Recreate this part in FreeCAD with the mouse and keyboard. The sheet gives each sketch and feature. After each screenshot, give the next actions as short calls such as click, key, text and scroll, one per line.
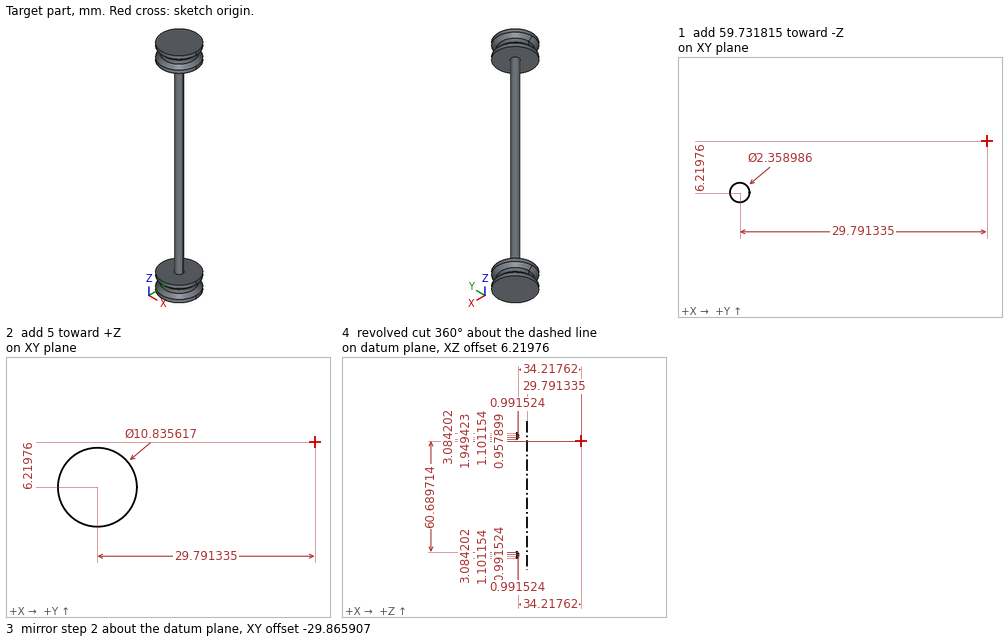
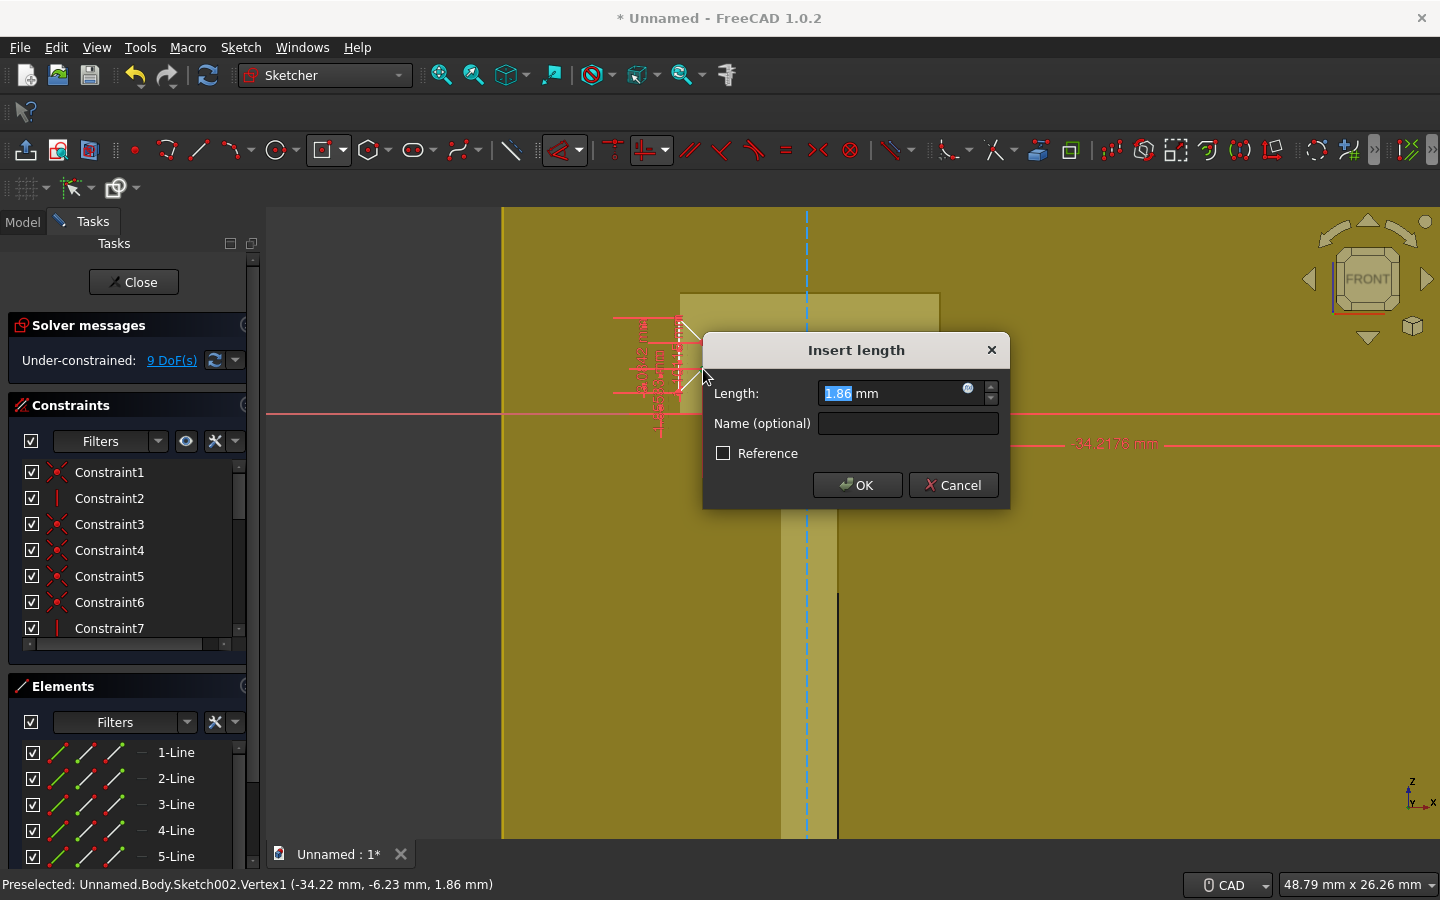
text(1.949423)
key(Return)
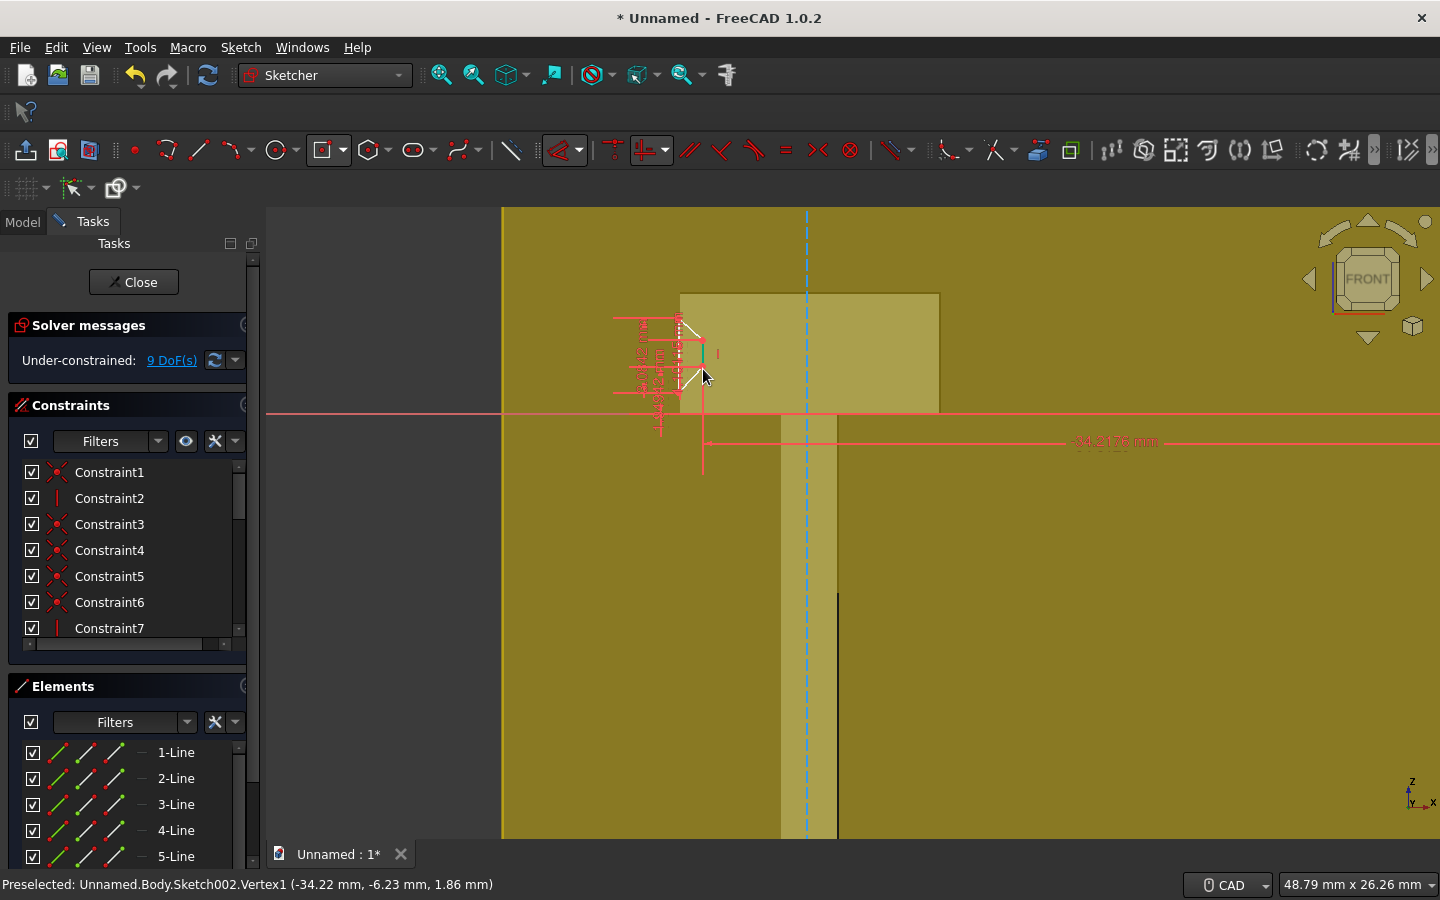
scroll(679, 393, up, 3)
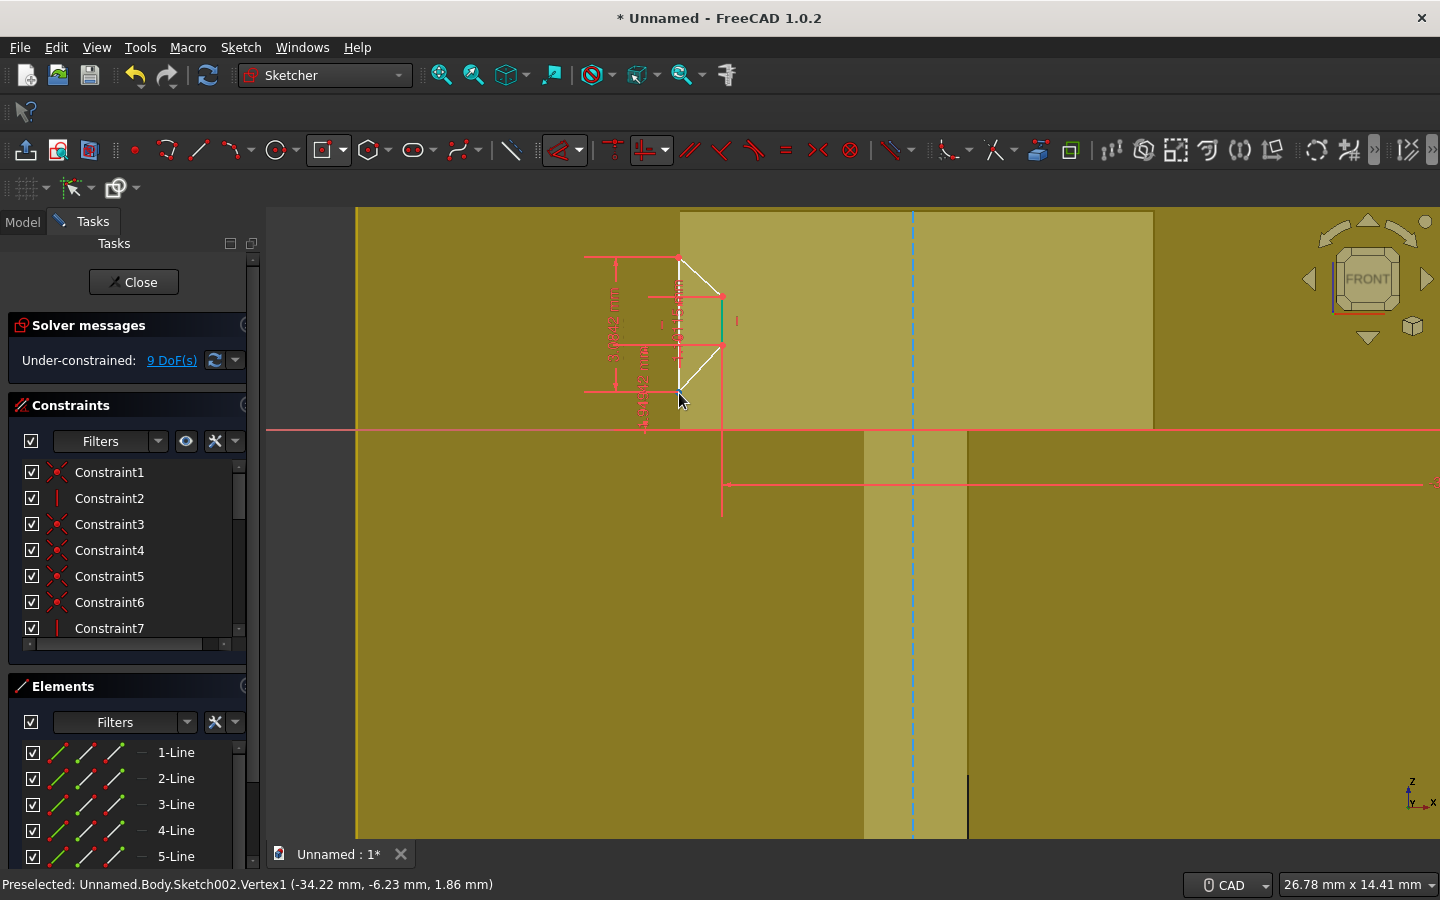
click(679, 392)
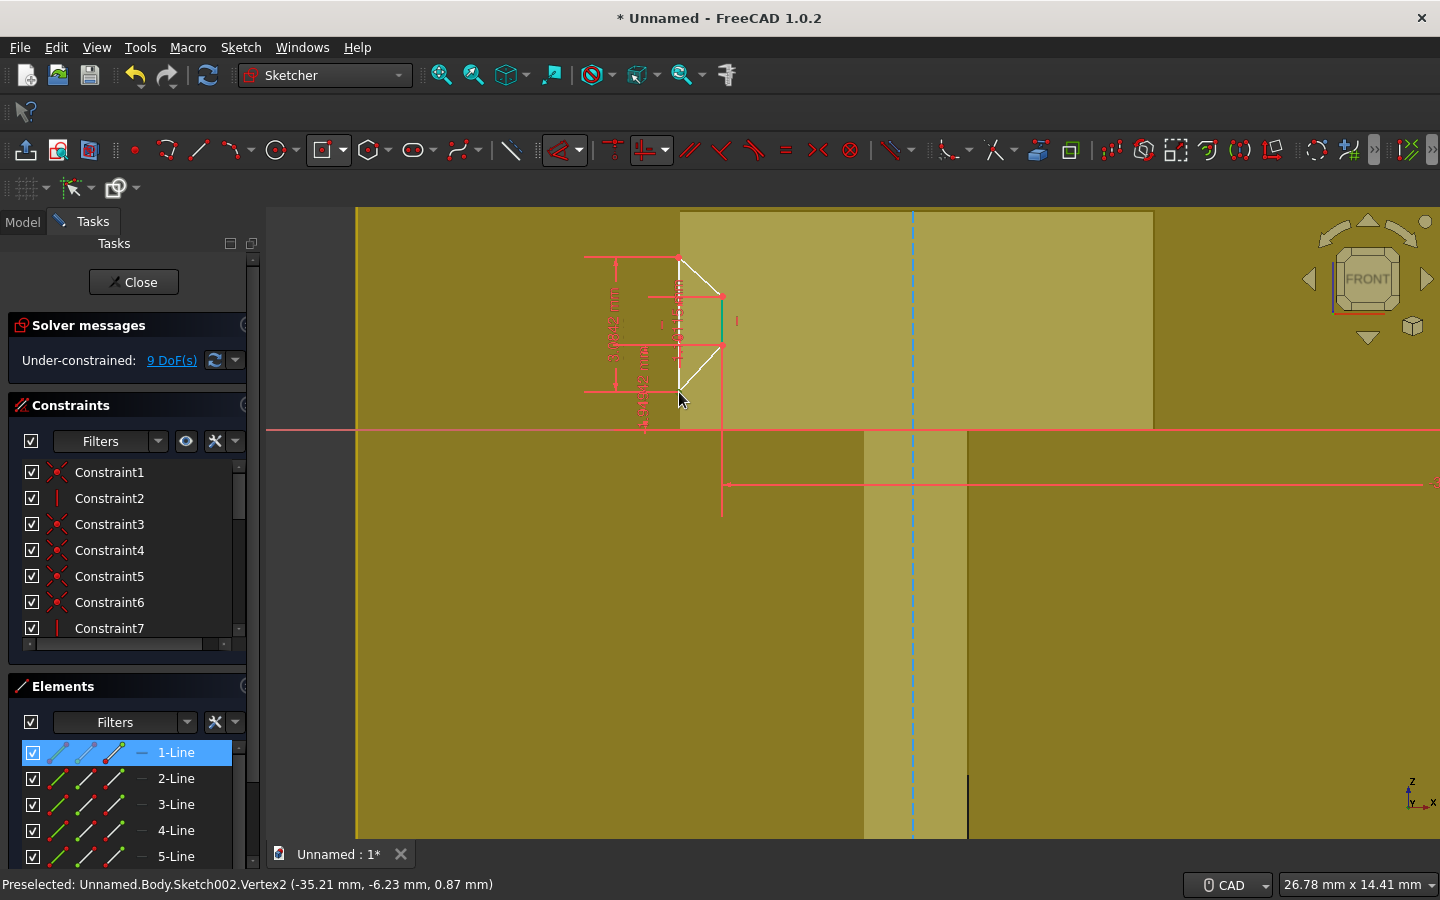
key(i)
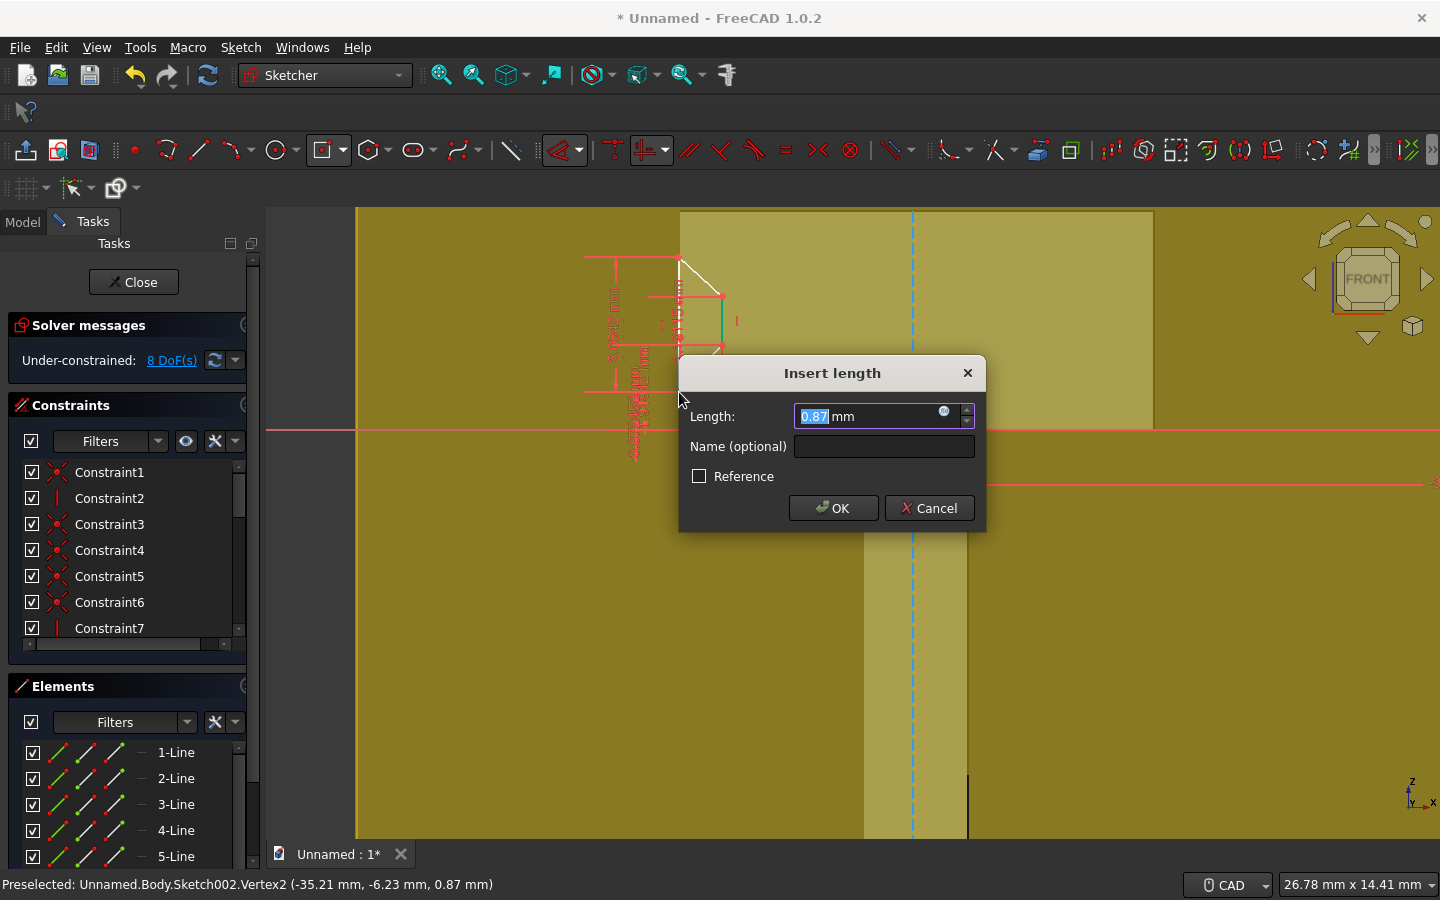
text(0.957899)
key(Return)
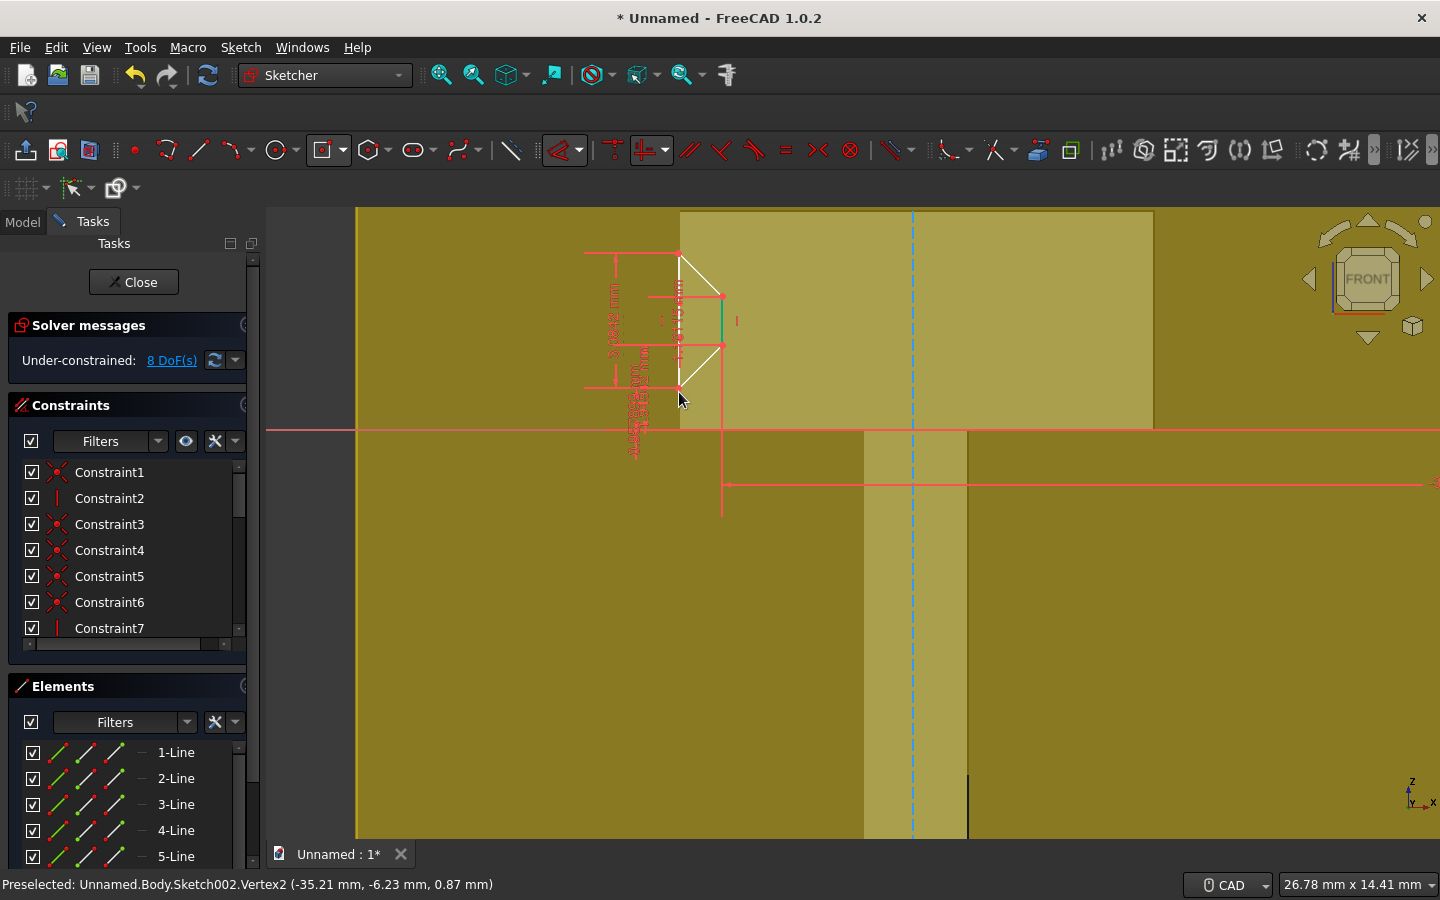
scroll(702, 371, down, 11)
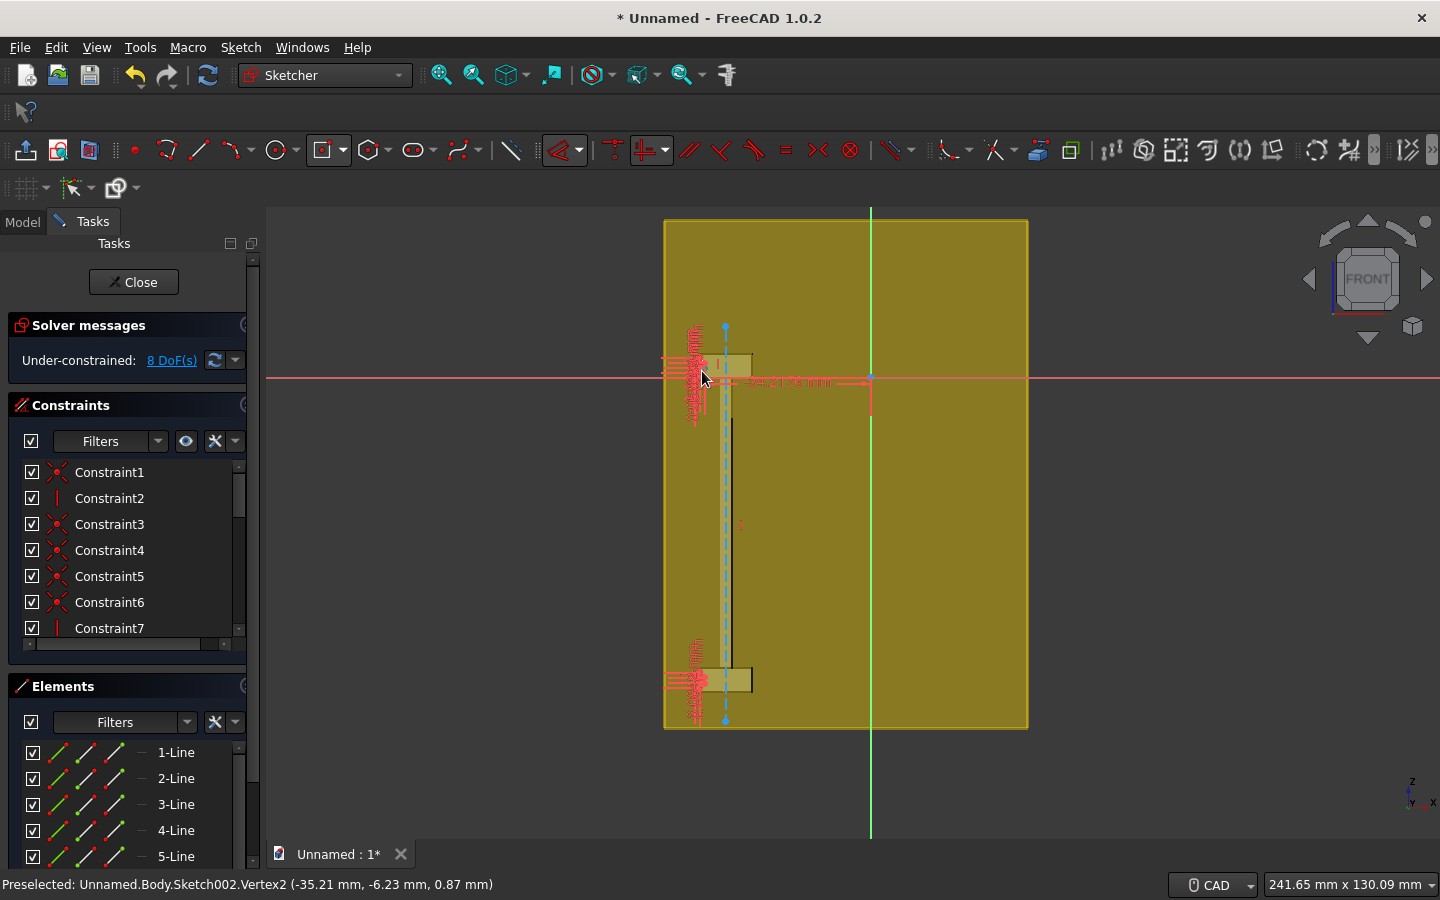
scroll(704, 678, up, 5)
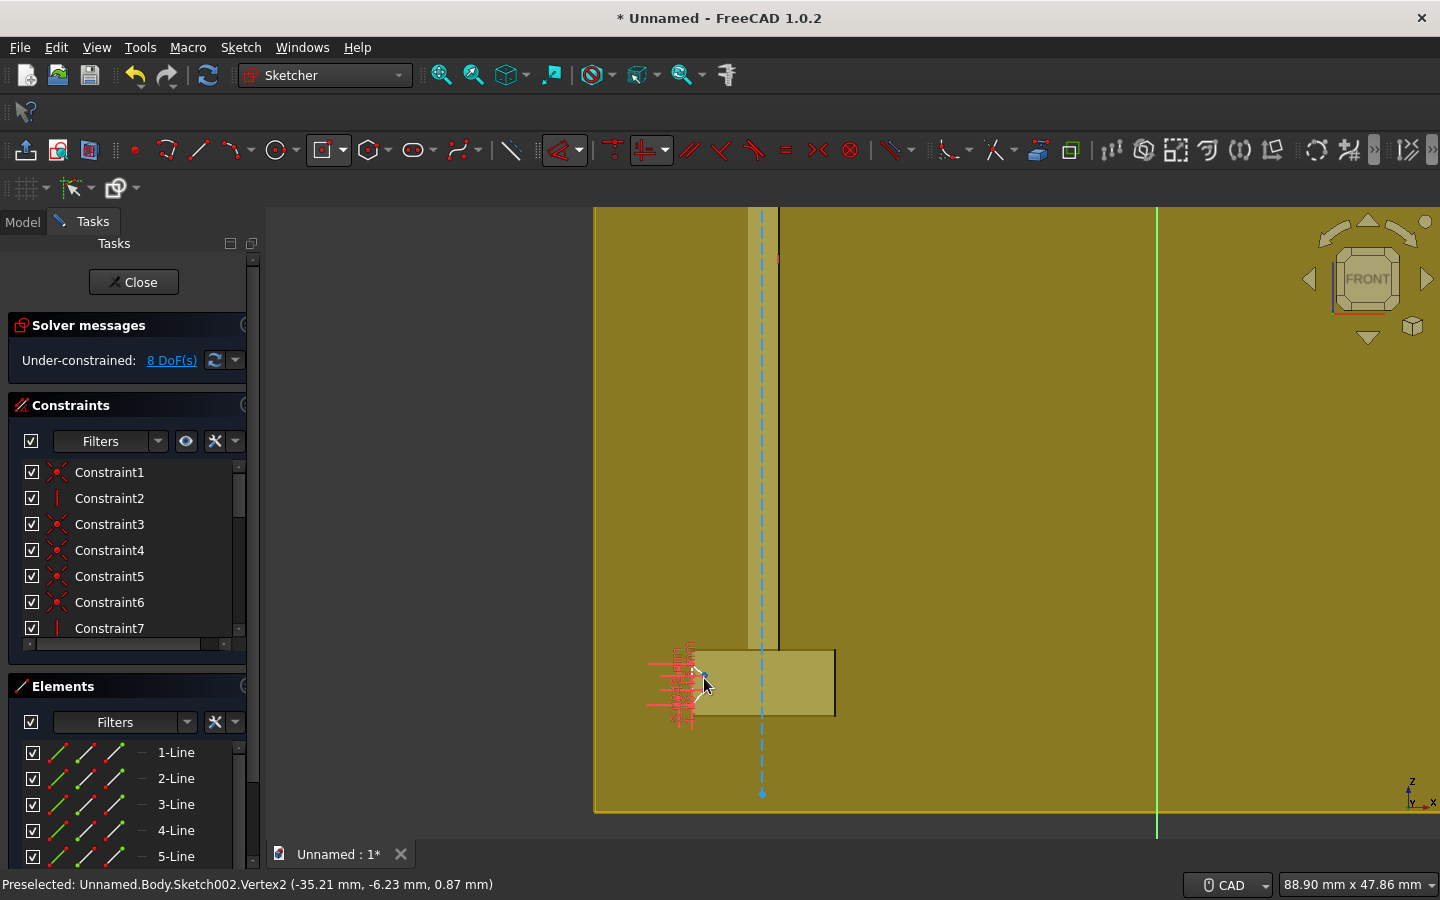
click(705, 676)